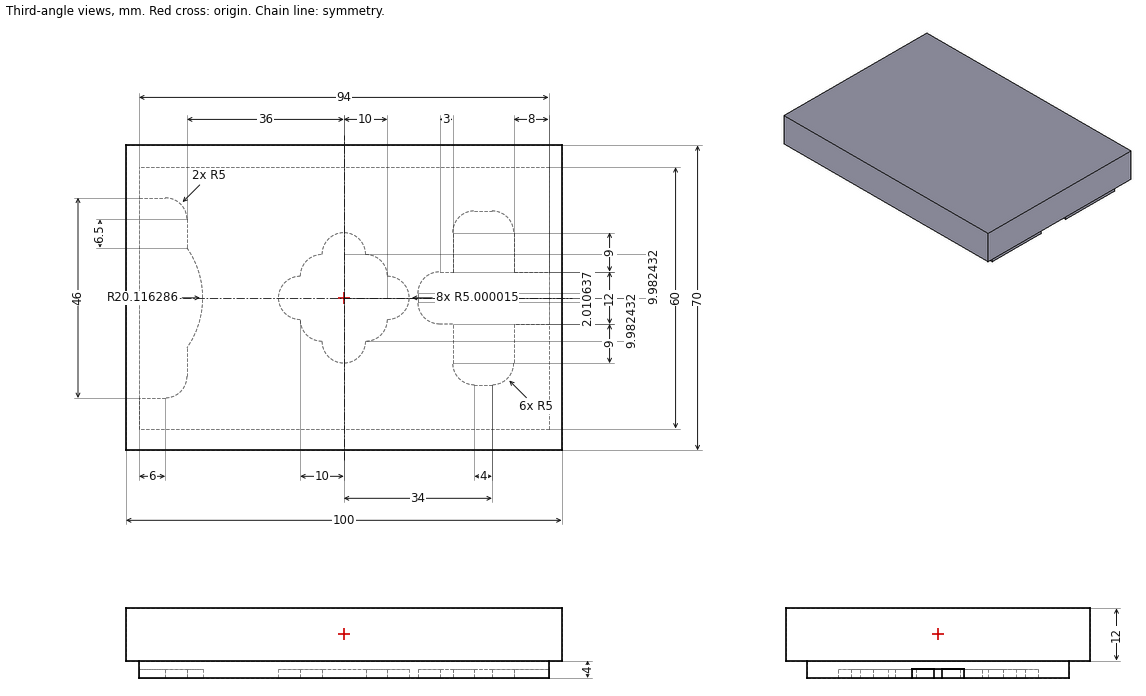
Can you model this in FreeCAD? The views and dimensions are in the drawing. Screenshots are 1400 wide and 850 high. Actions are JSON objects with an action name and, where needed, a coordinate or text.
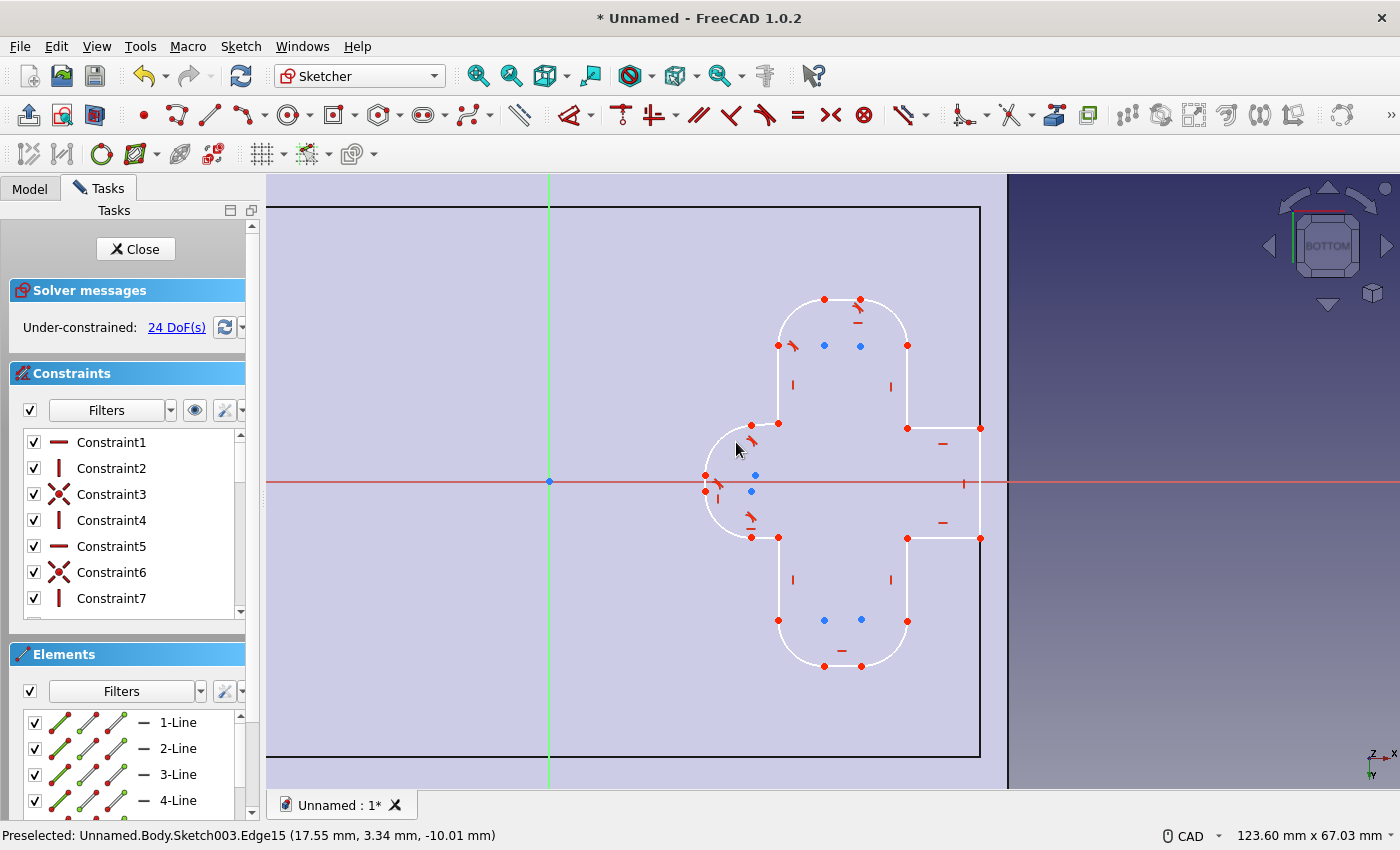
{"action": "left_click", "coordinate": [779, 563]}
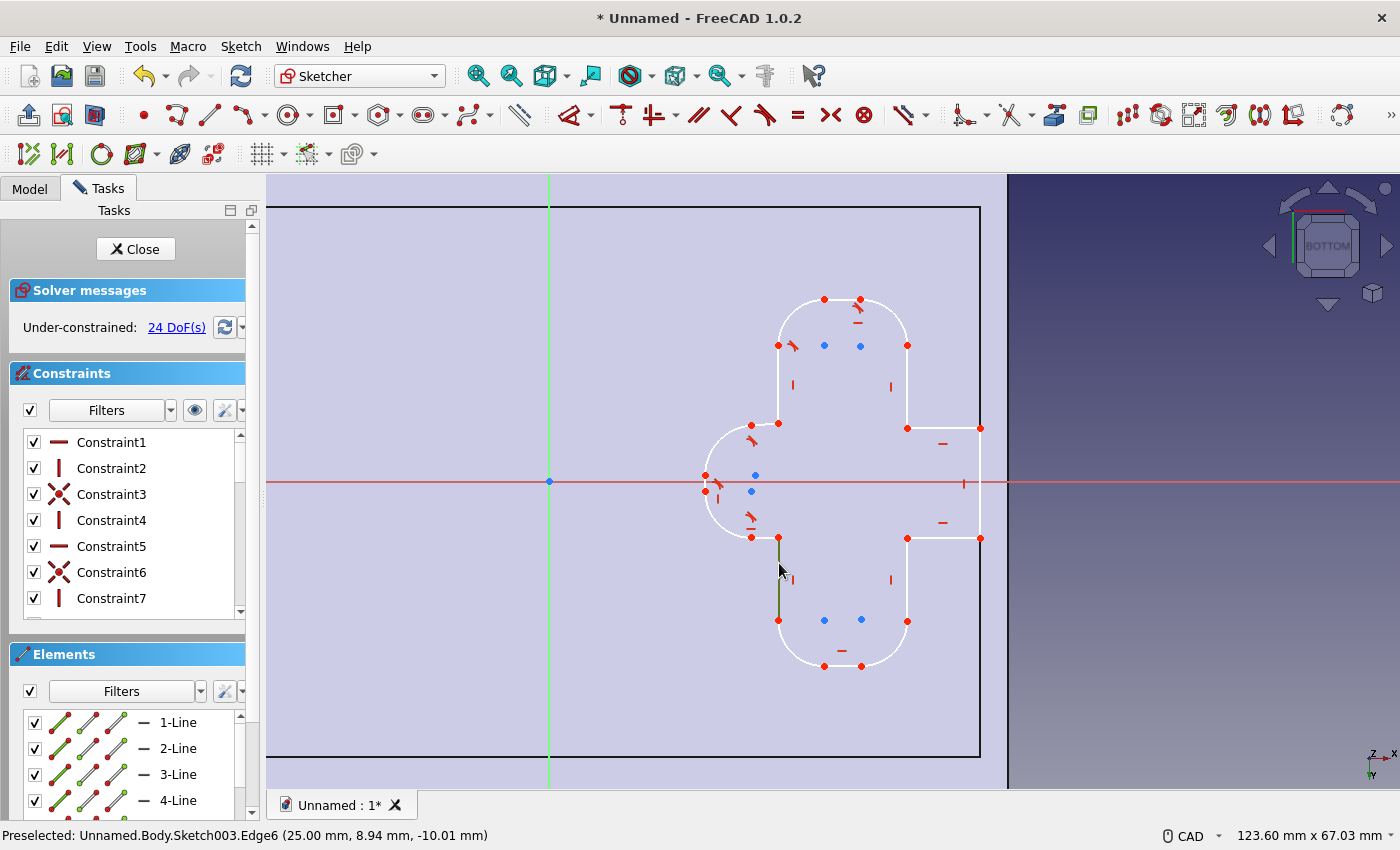
{"action": "left_click", "coordinate": [783, 641]}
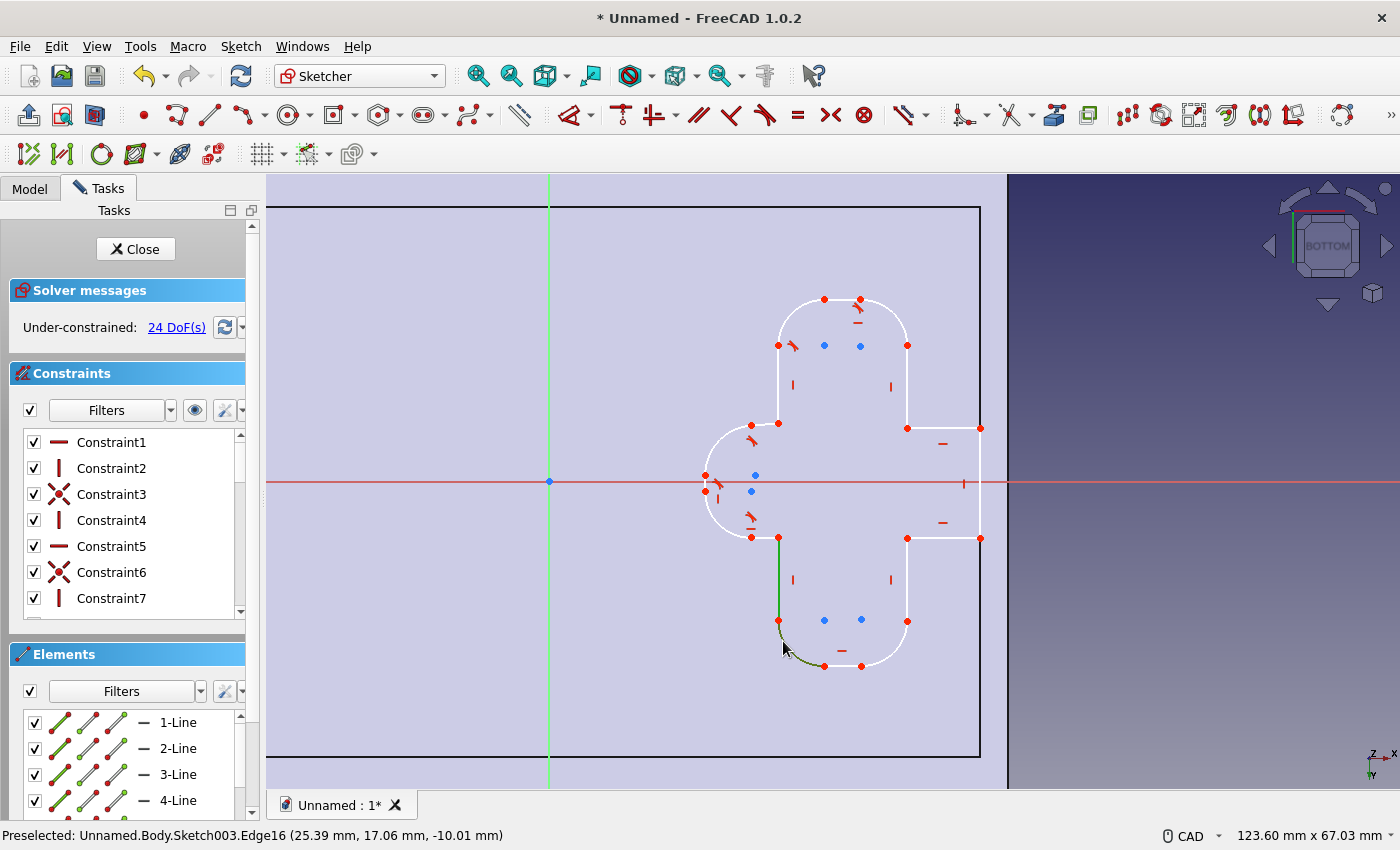
{"action": "left_click", "coordinate": [765, 116]}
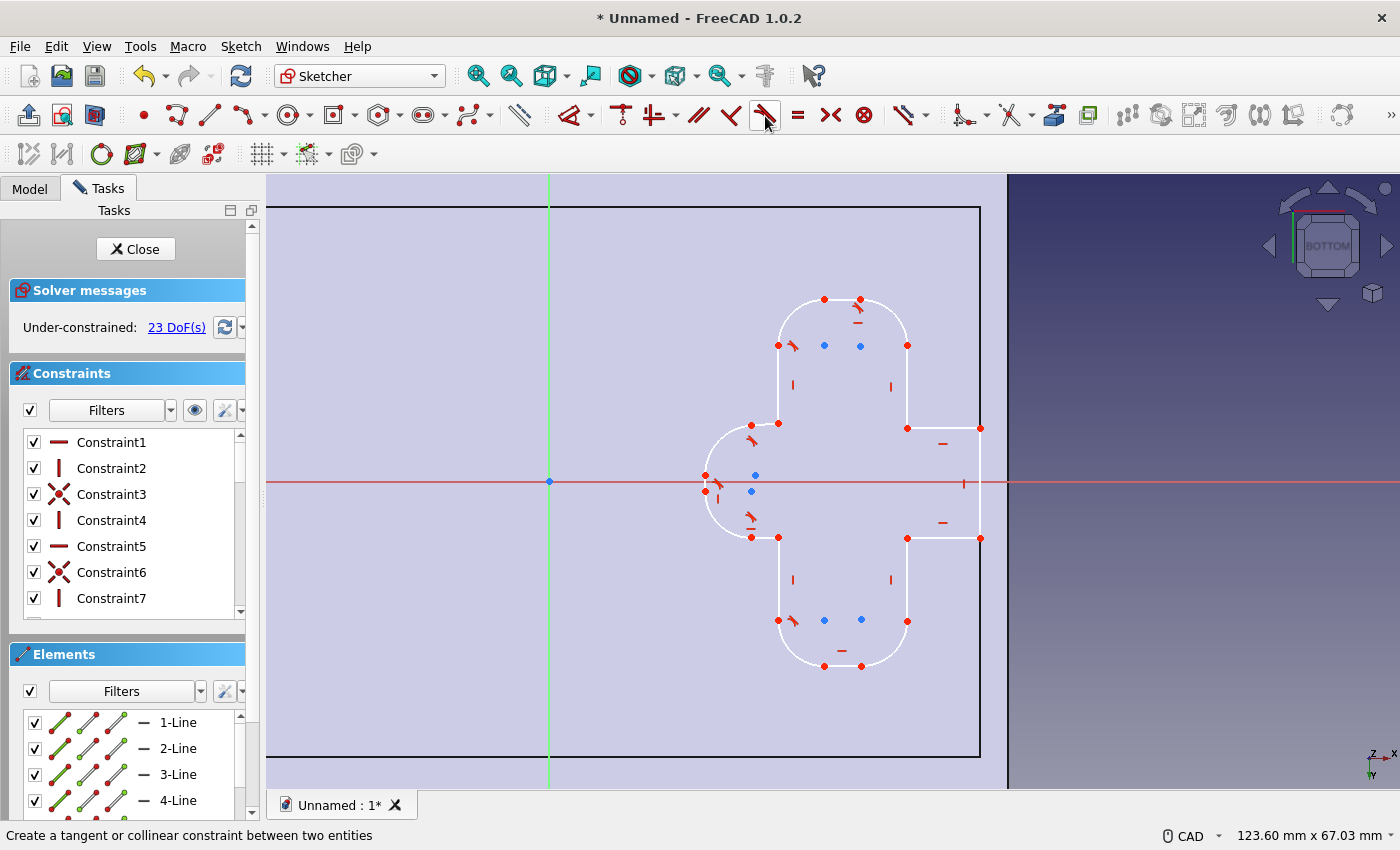
{"action": "scroll", "coordinate": [835, 666], "scroll_direction": "up", "scroll_amount": 2}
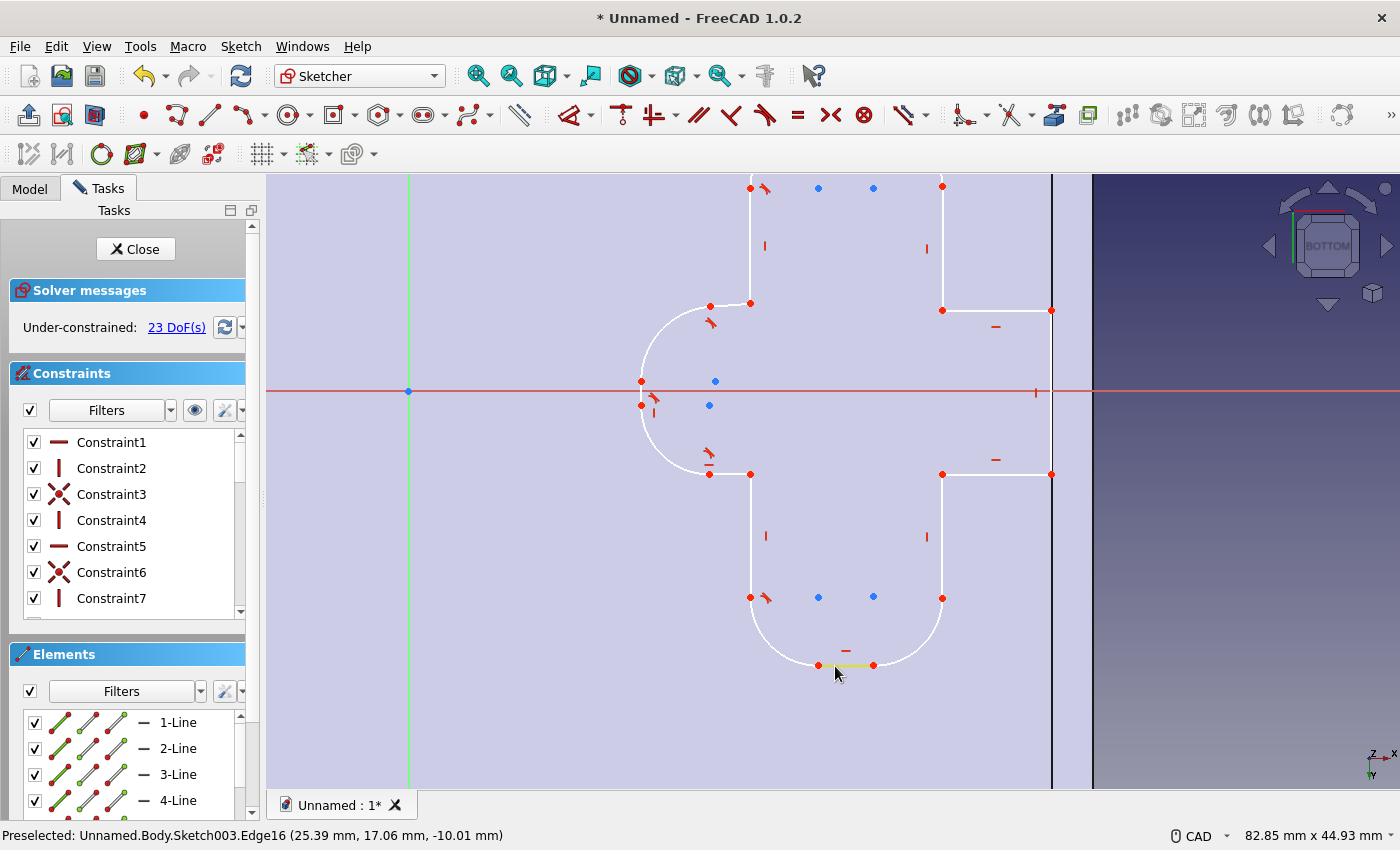
{"action": "left_click", "coordinate": [835, 666]}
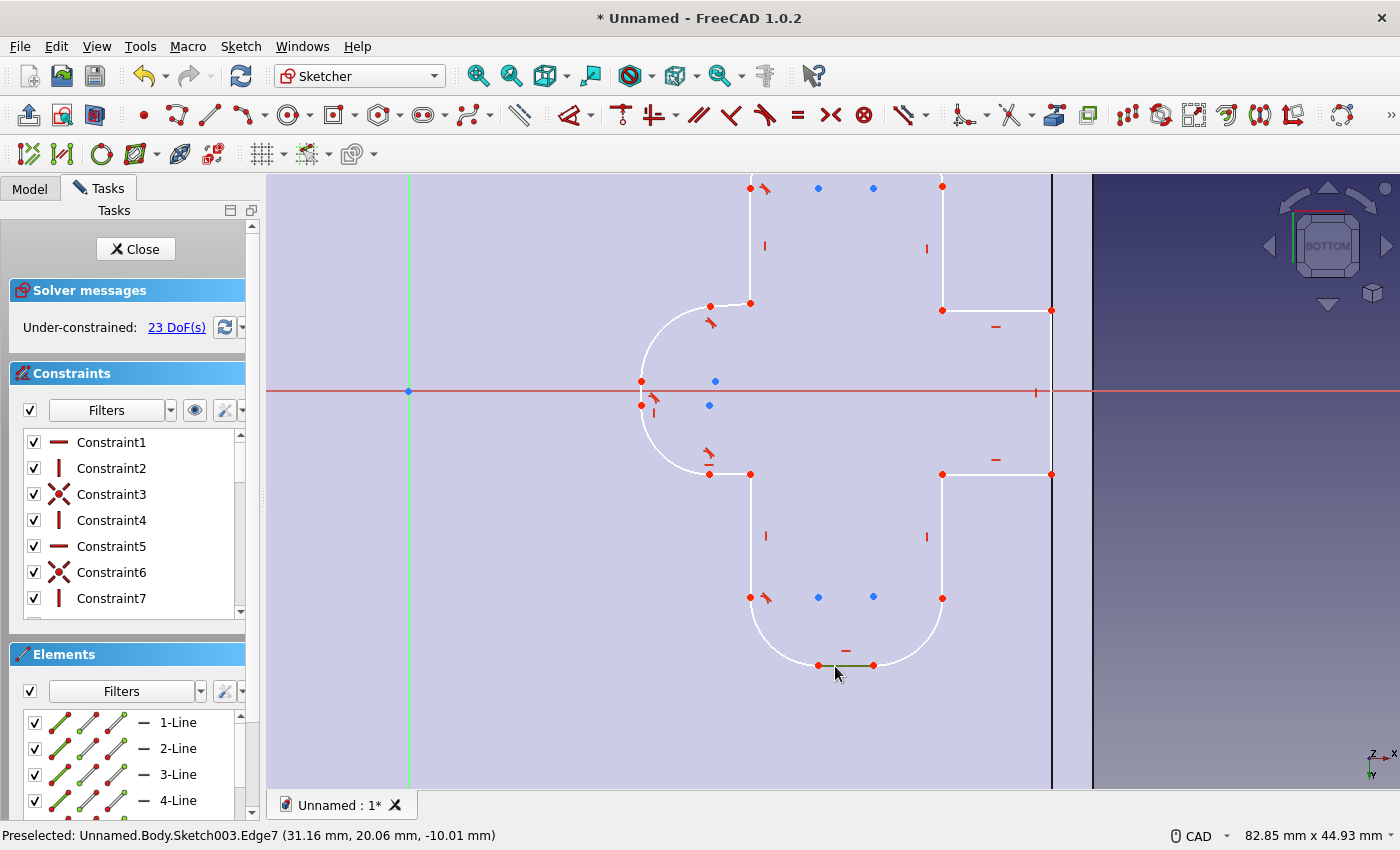
{"action": "left_click", "coordinate": [758, 628]}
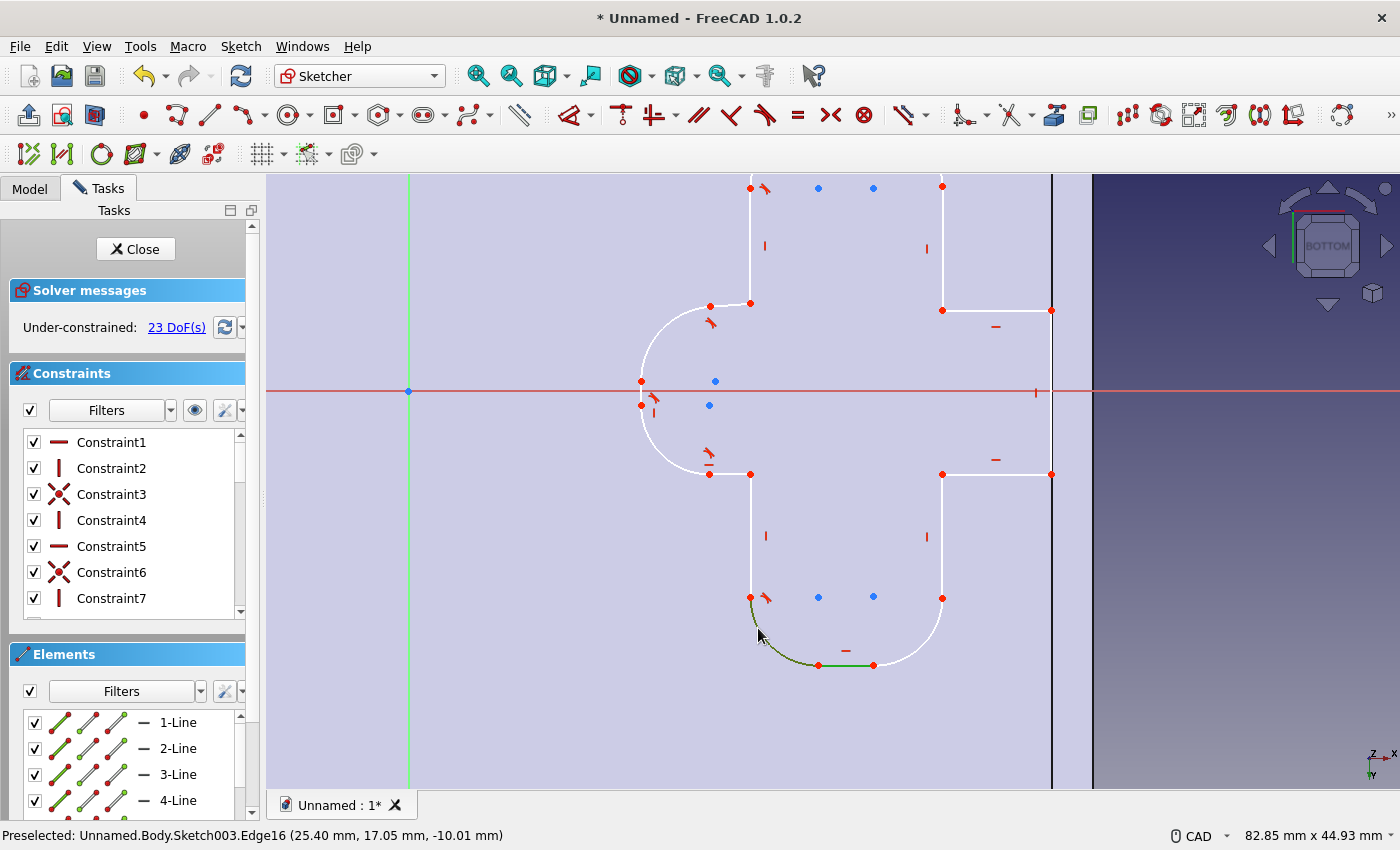
{"action": "left_click", "coordinate": [765, 116]}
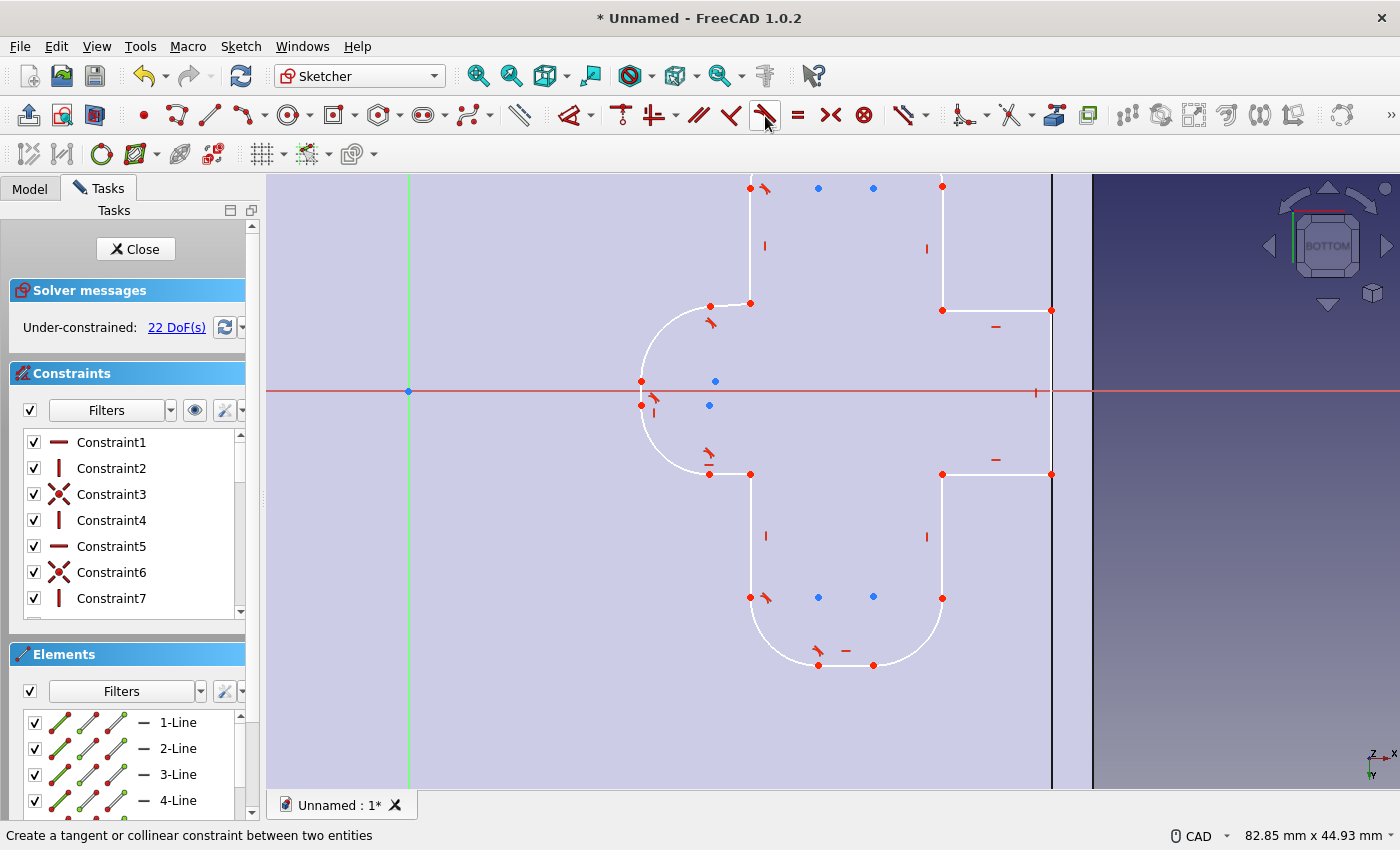
{"action": "left_click", "coordinate": [835, 666]}